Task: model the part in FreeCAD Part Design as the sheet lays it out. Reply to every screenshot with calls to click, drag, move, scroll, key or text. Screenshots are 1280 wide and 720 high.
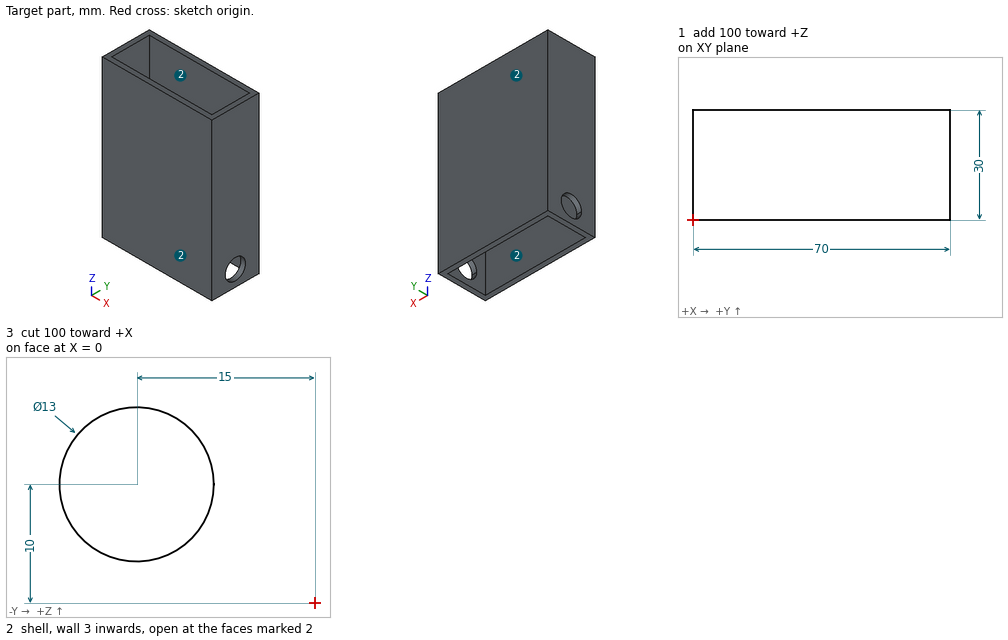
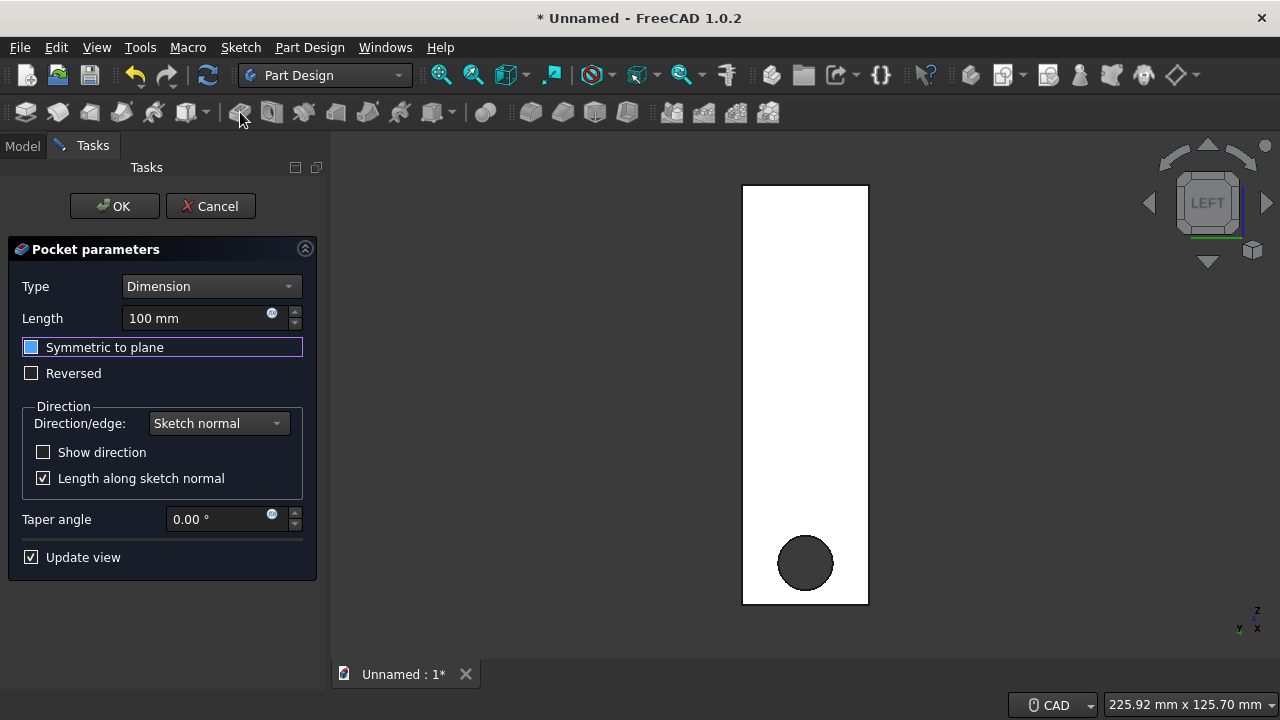
click(115, 206)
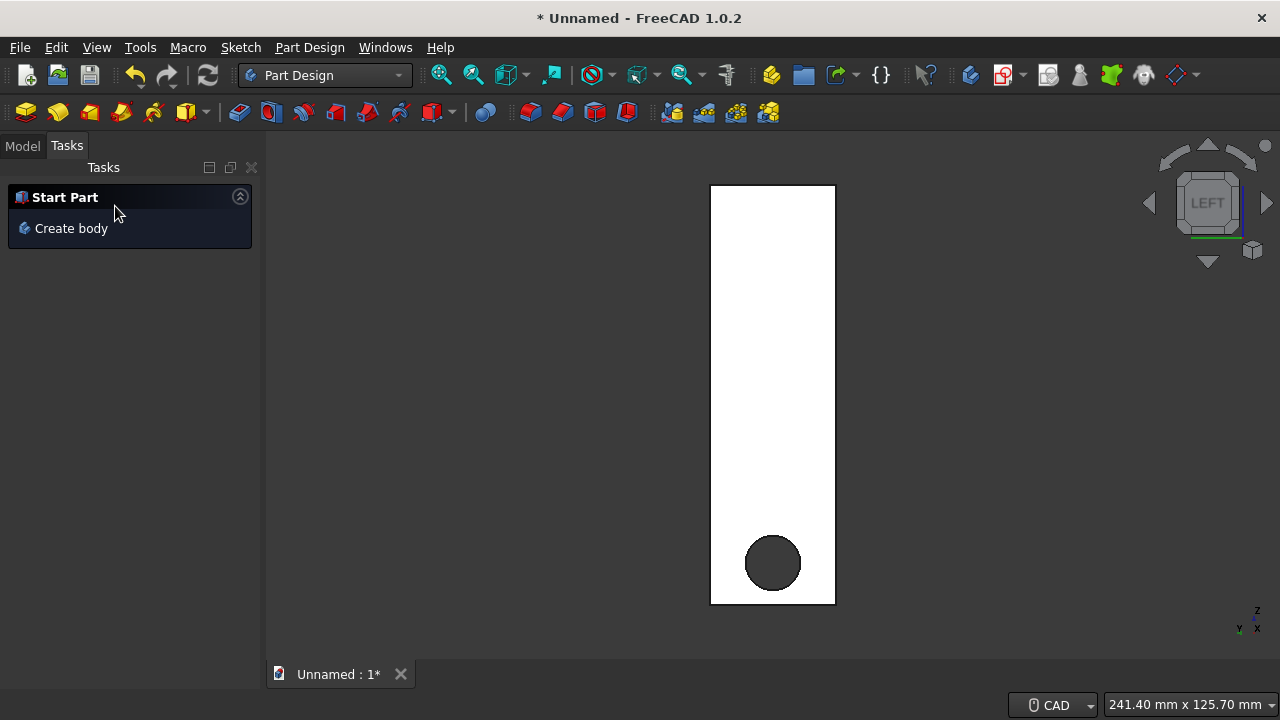
key(0)